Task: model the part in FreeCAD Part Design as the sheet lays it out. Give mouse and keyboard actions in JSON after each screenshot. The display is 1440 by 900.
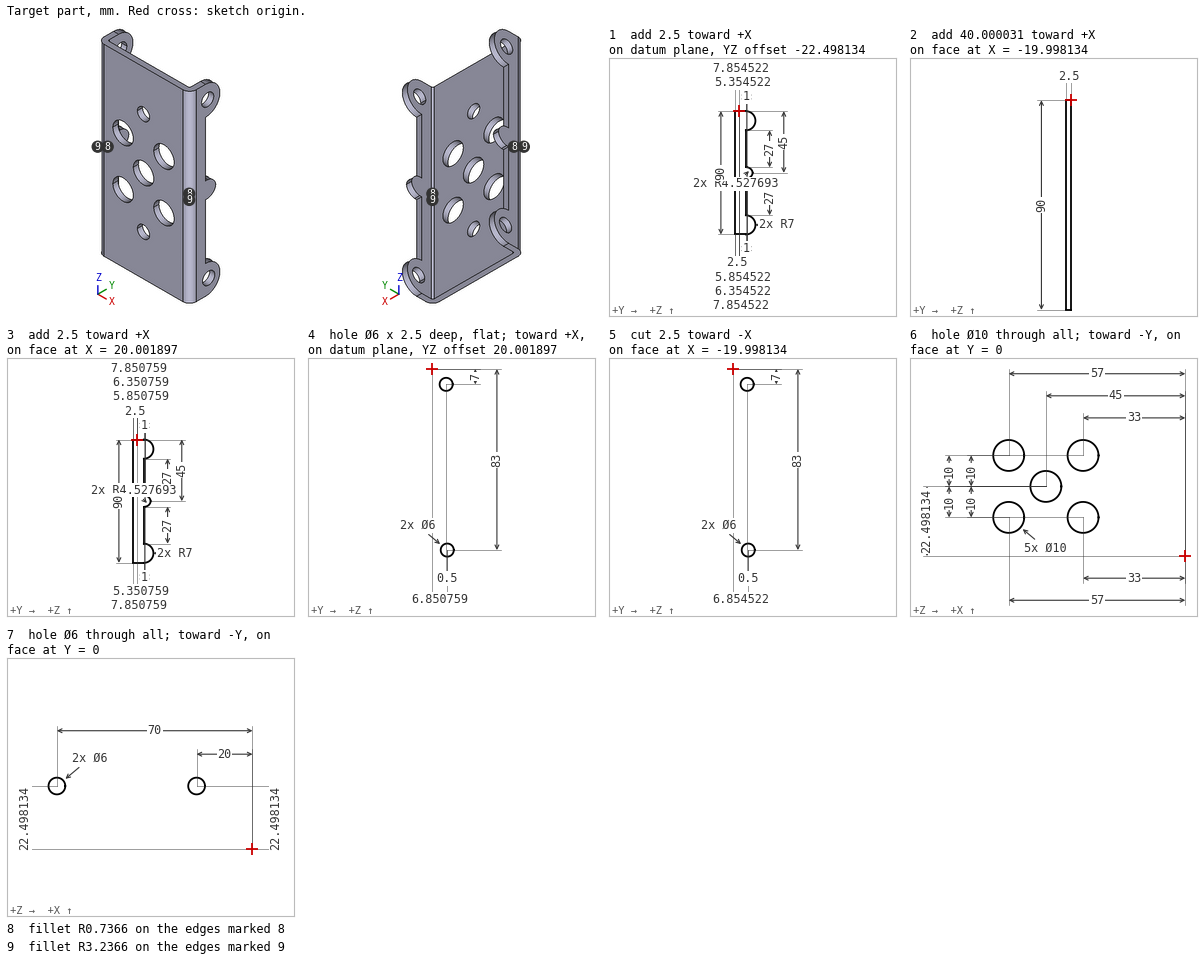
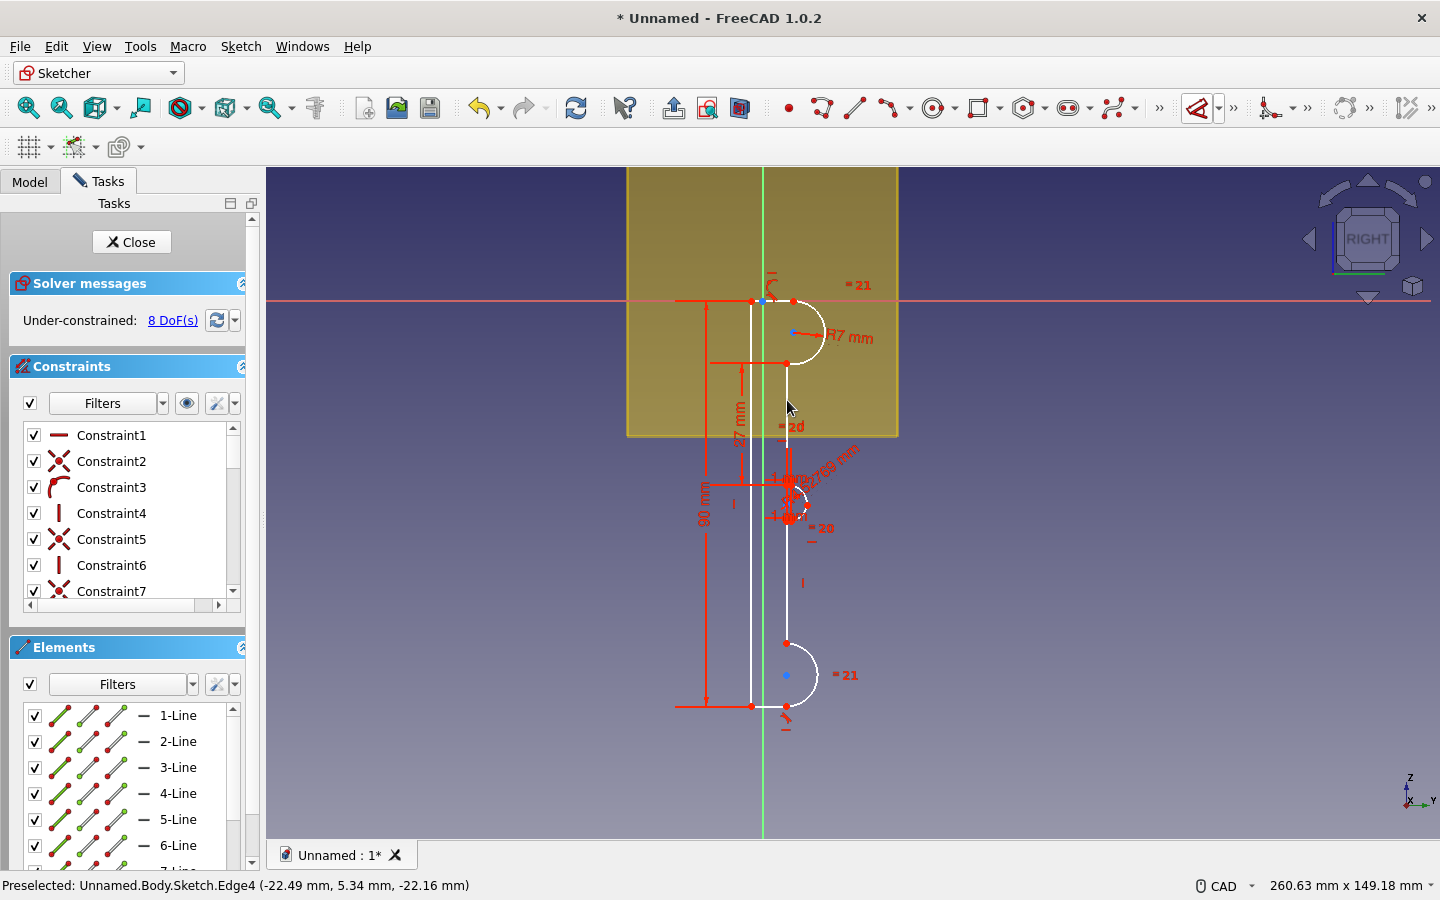
{"action": "left_click", "coordinate": [787, 558]}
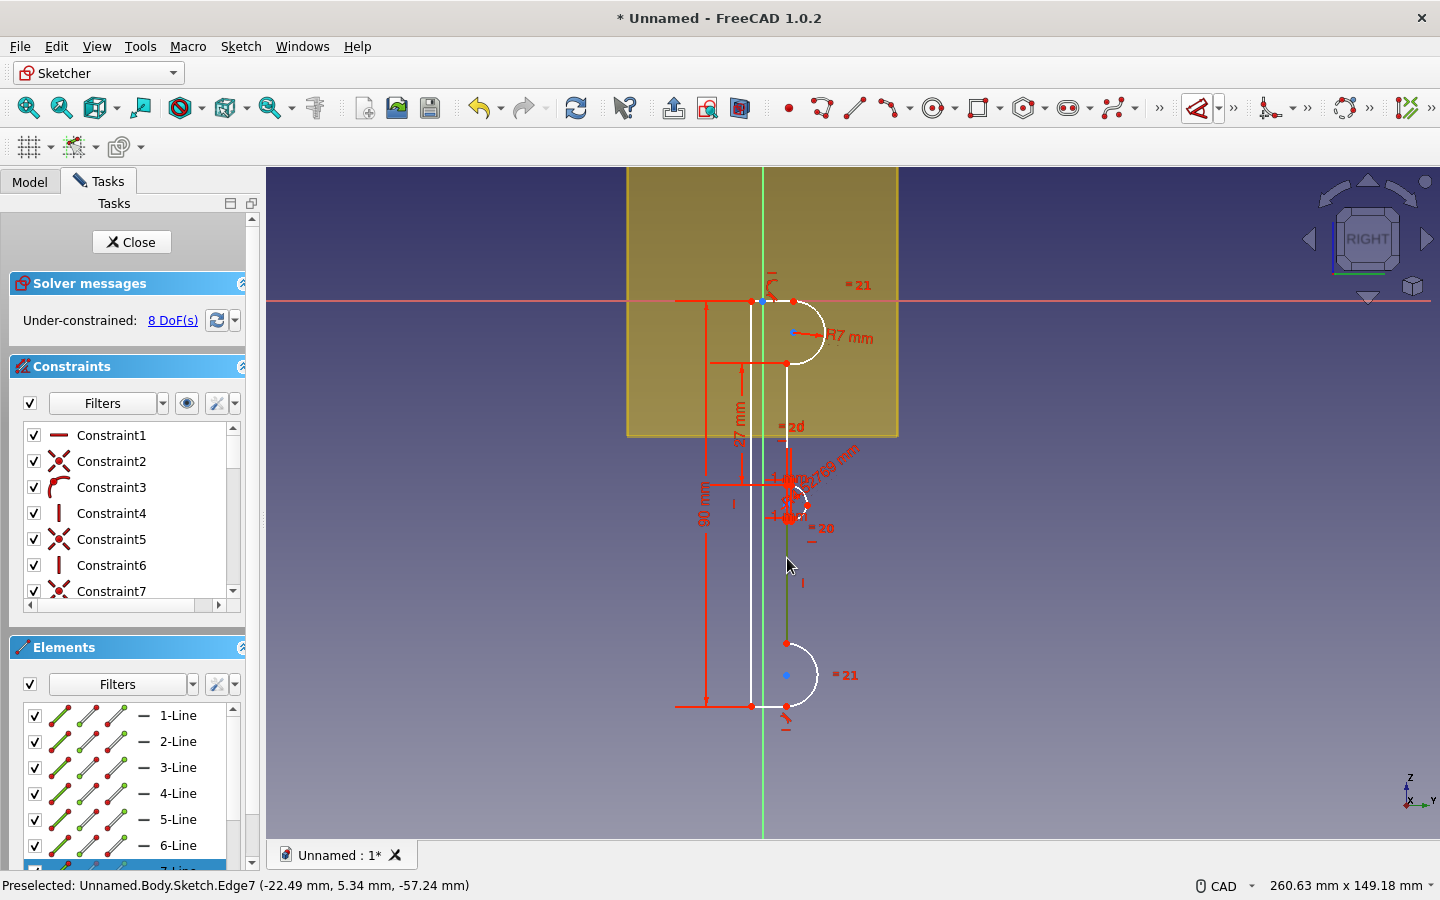
{"action": "left_click", "coordinate": [1218, 108]}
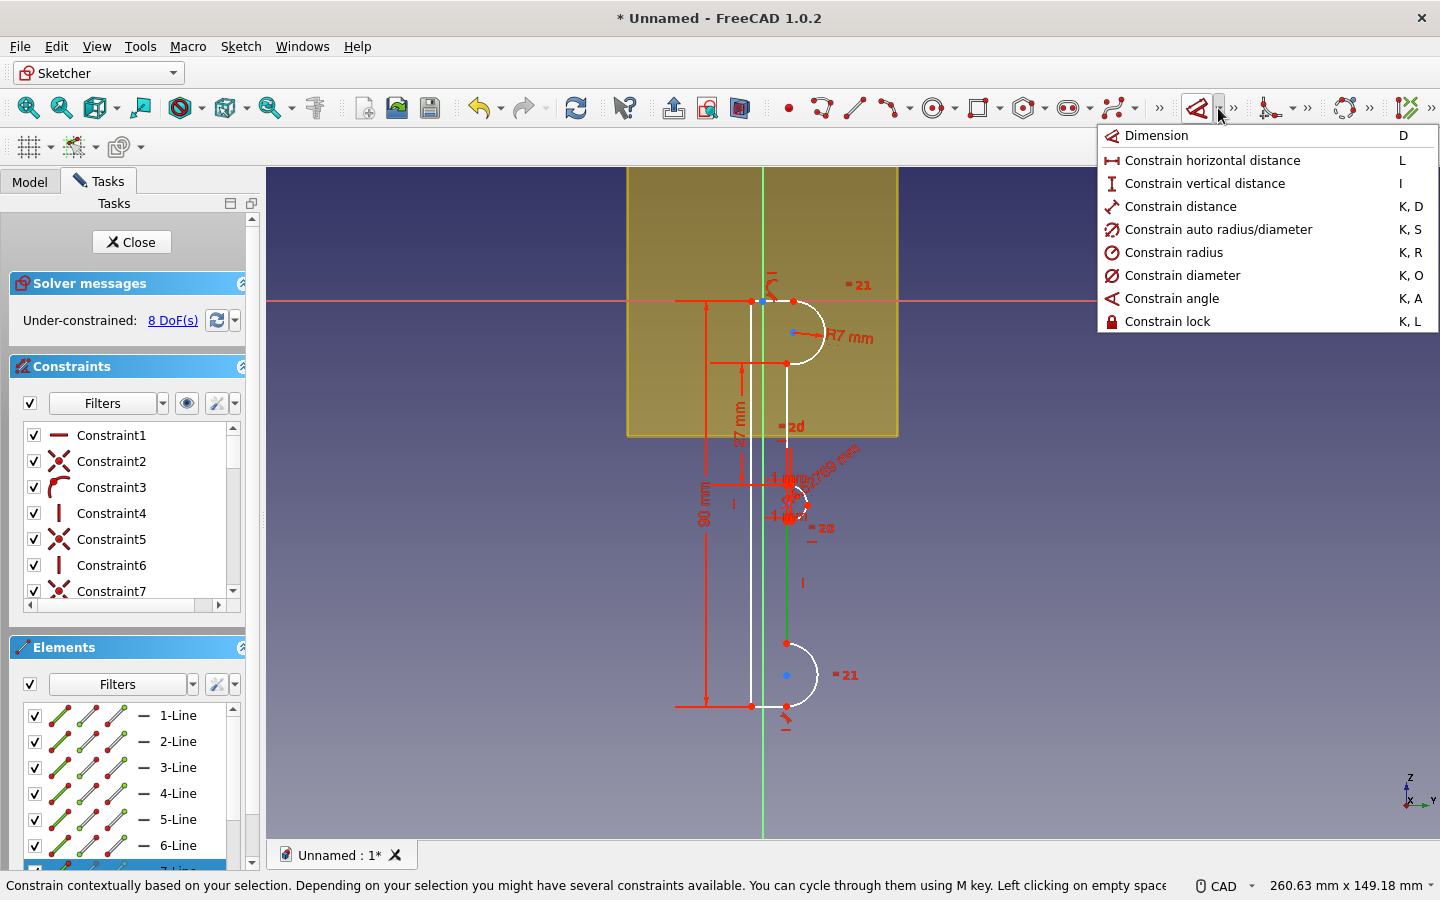
{"action": "left_click", "coordinate": [1268, 184]}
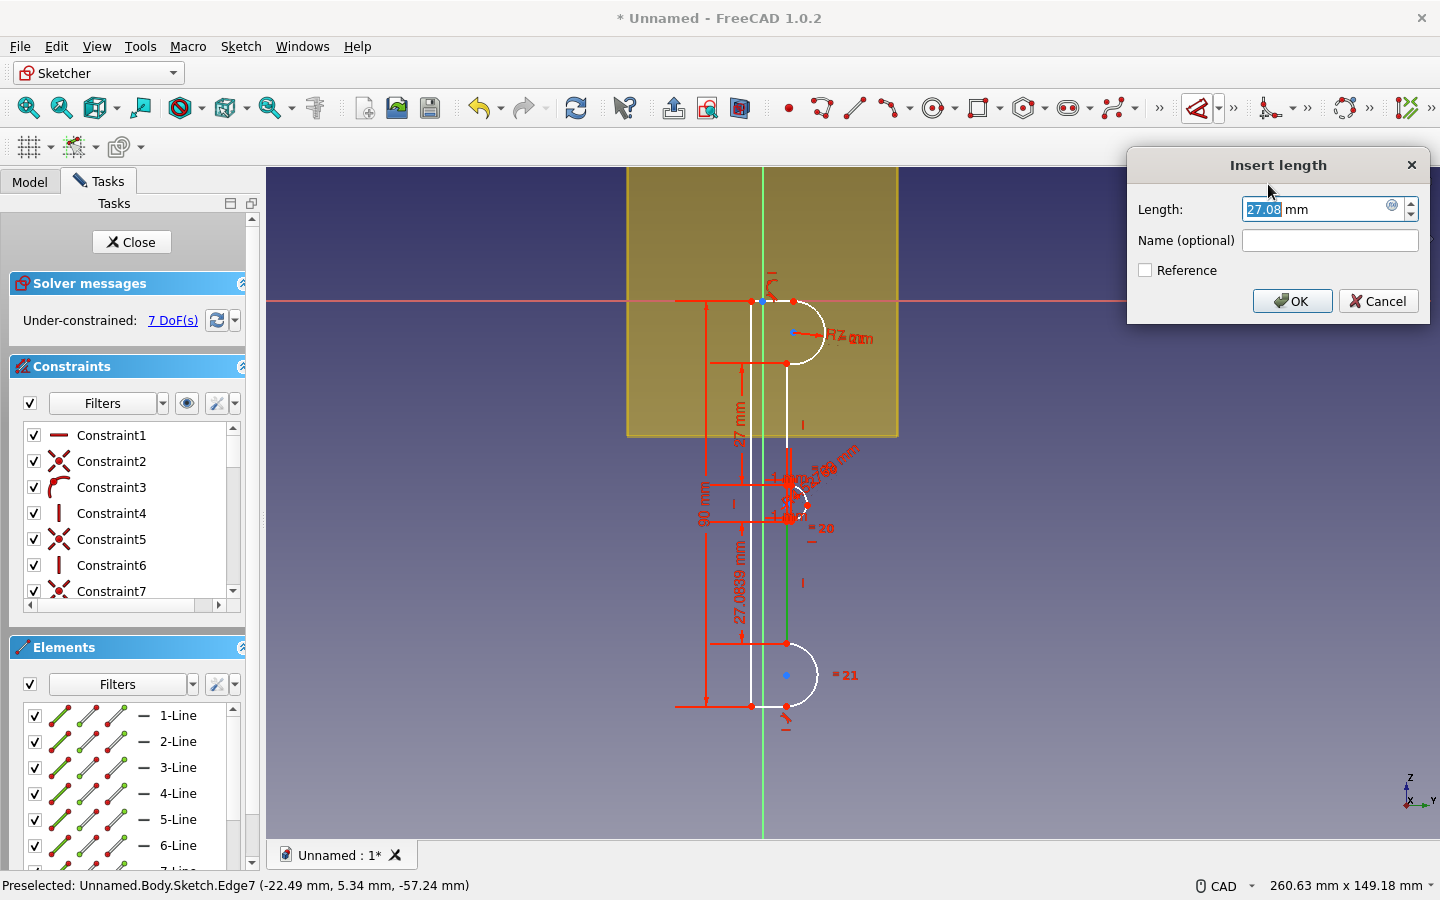
{"action": "type", "text": "27"}
{"action": "key", "text": "Return"}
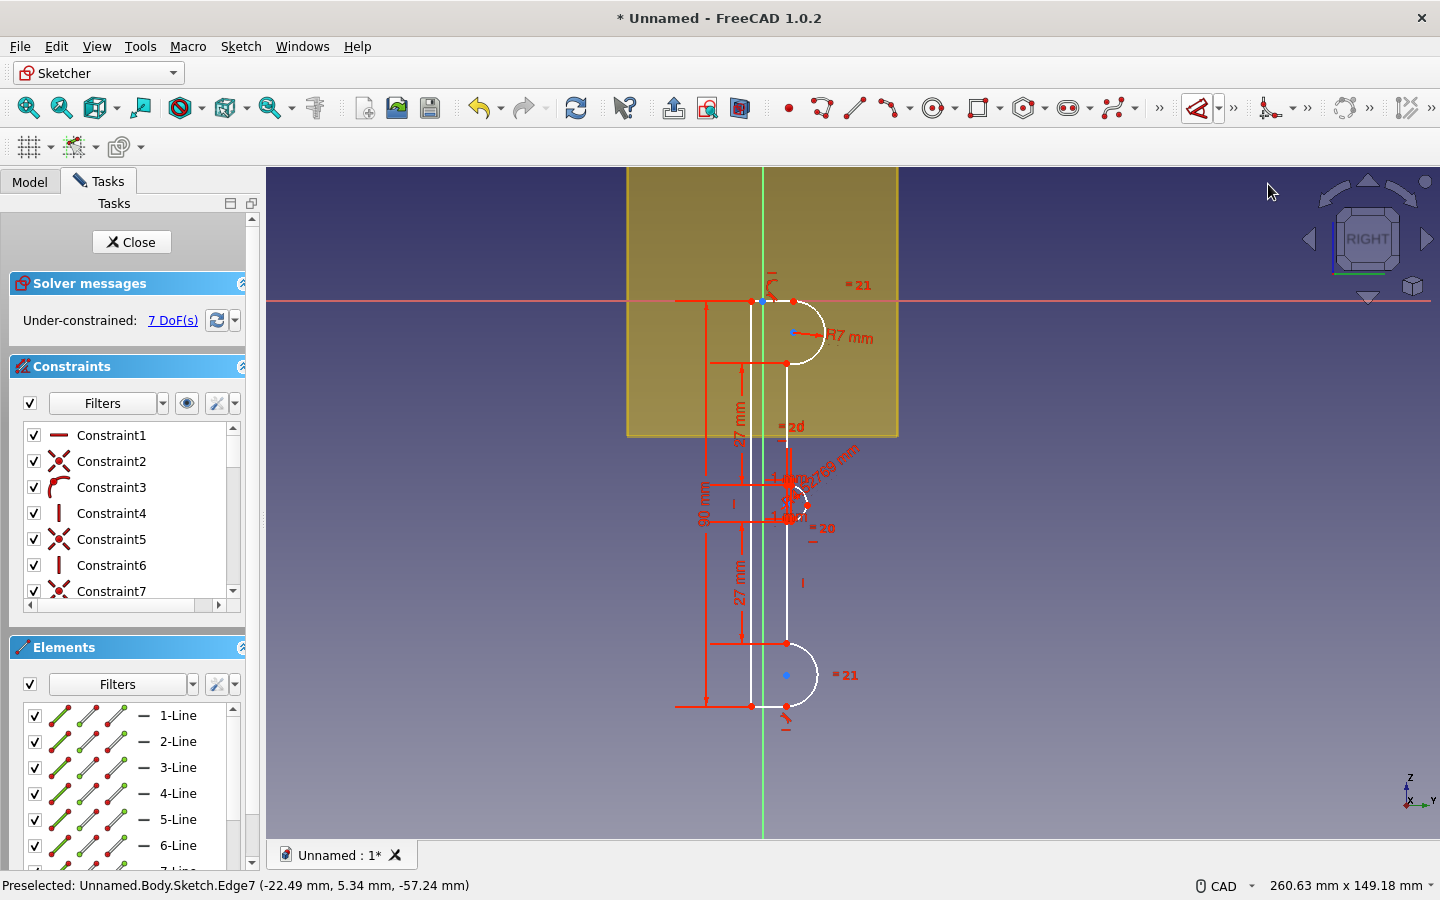
{"action": "left_click", "coordinate": [807, 505]}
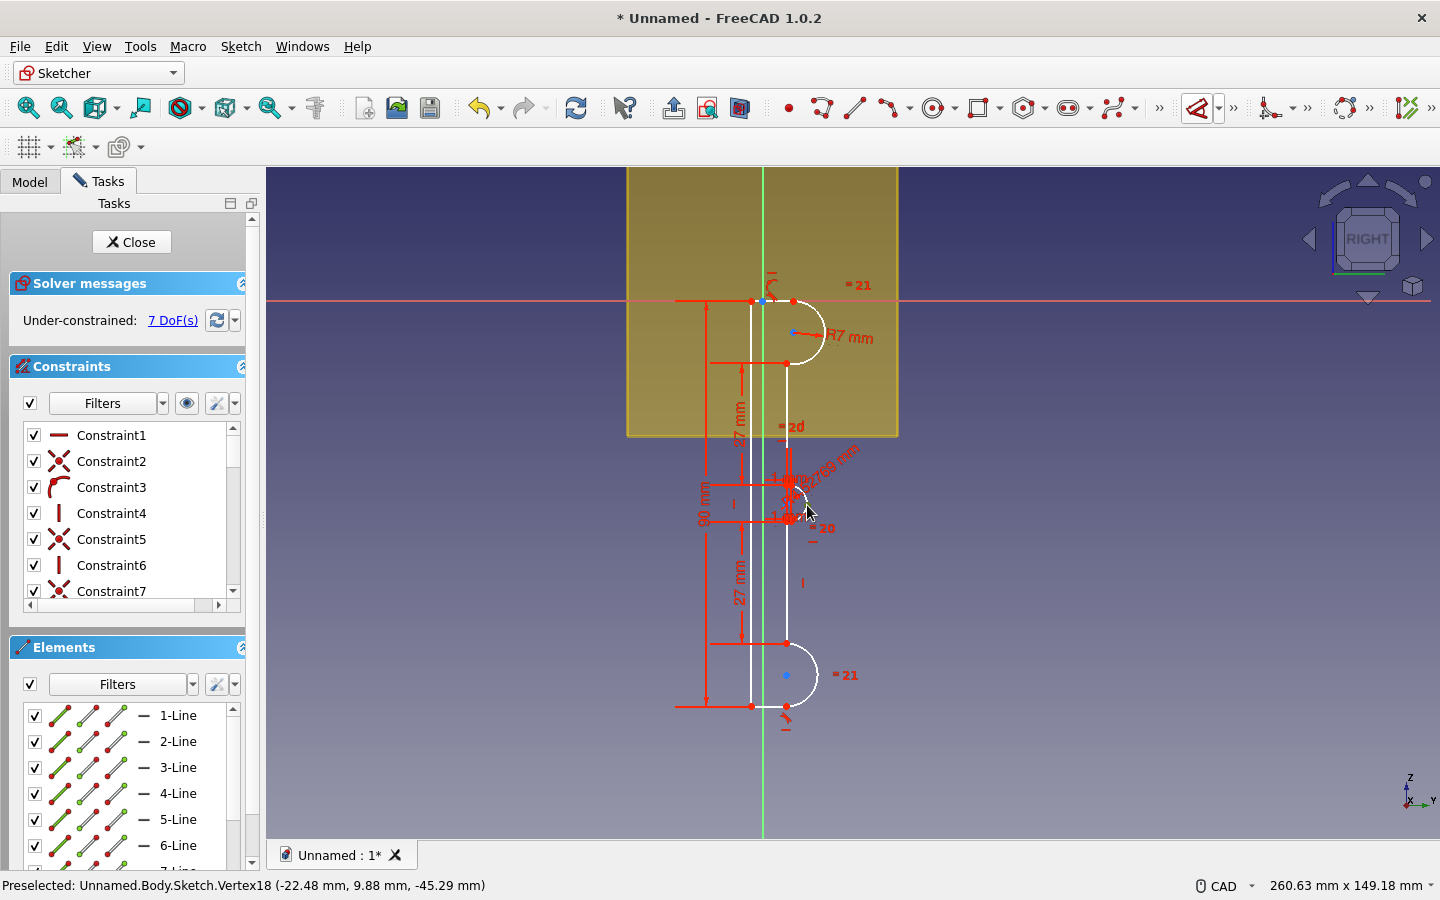
{"action": "left_click", "coordinate": [1218, 108]}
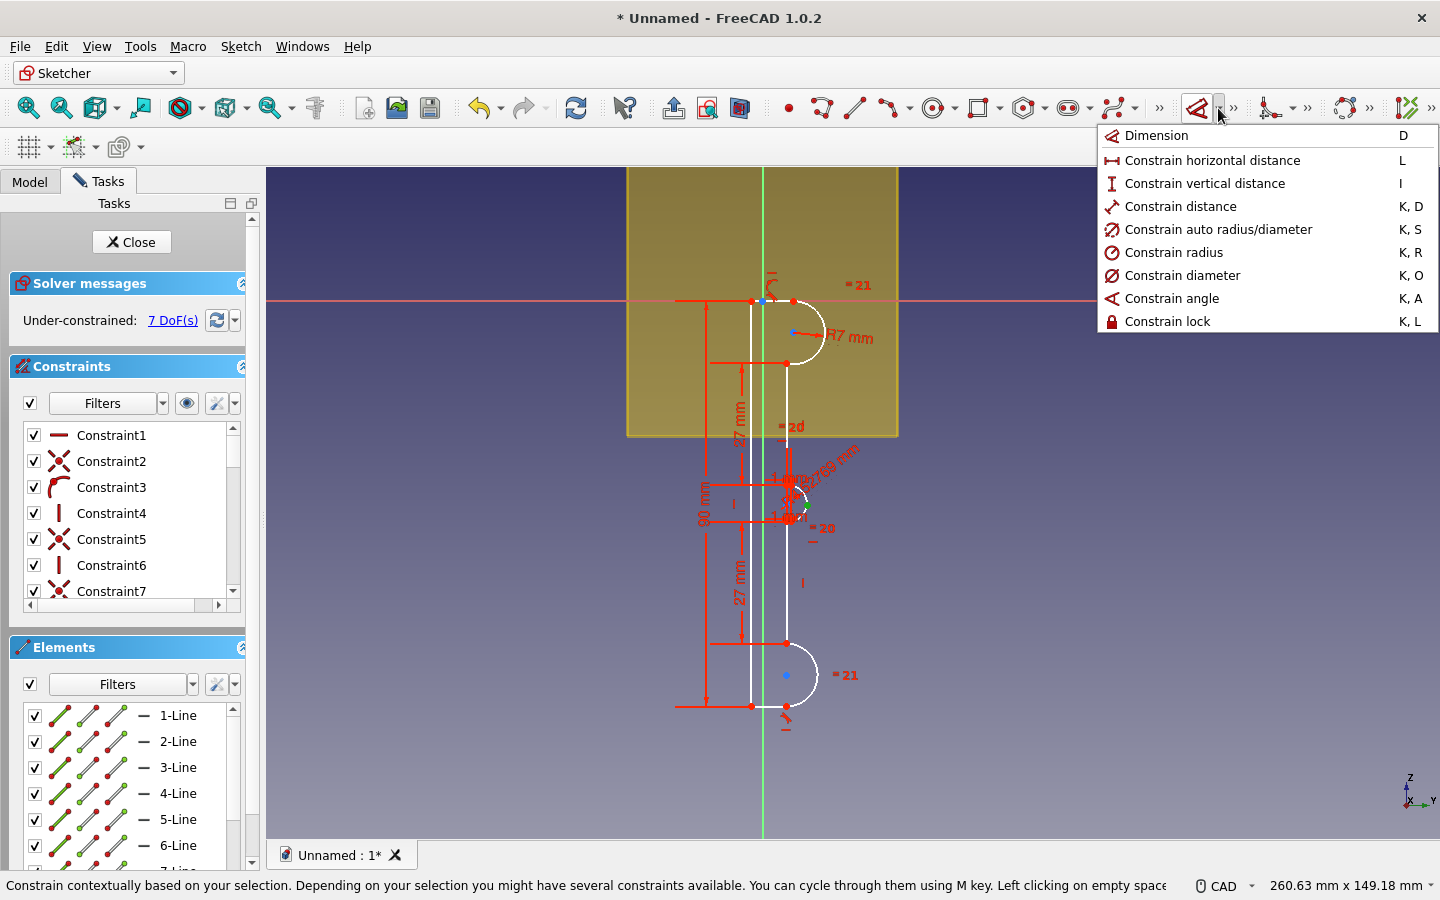
{"action": "left_click", "coordinate": [1268, 184]}